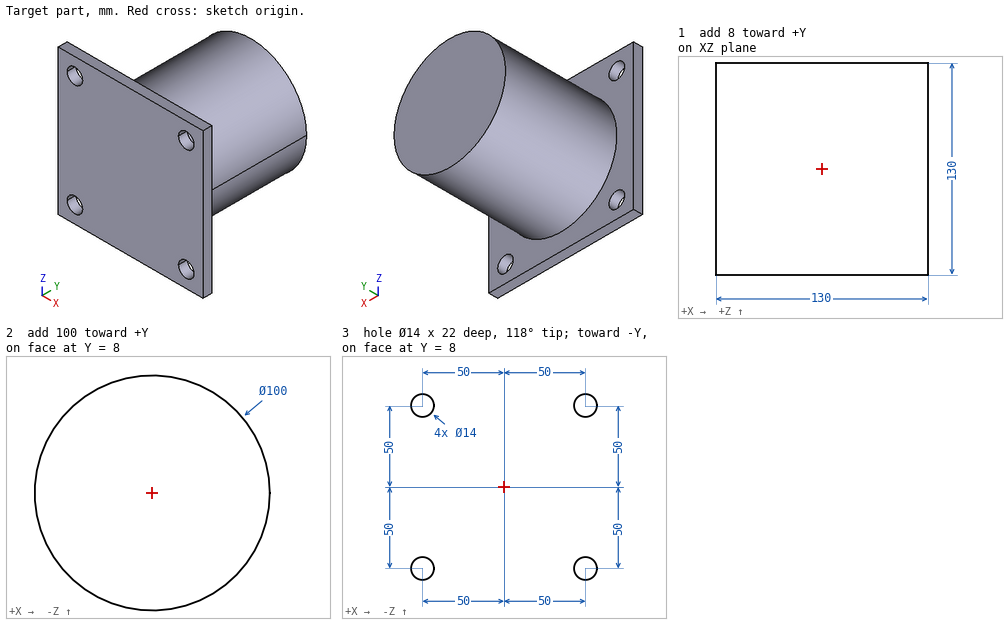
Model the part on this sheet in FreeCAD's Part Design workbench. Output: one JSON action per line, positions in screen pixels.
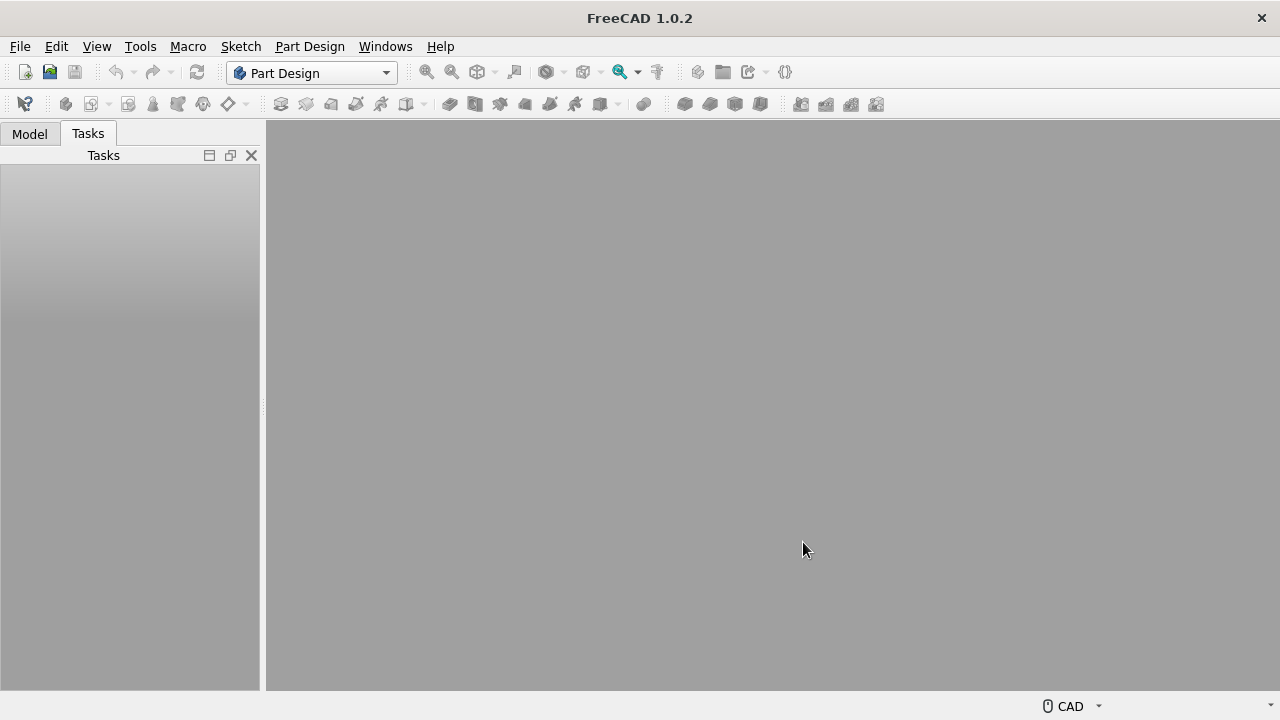
{"action": "left_click", "coordinate": [25, 72]}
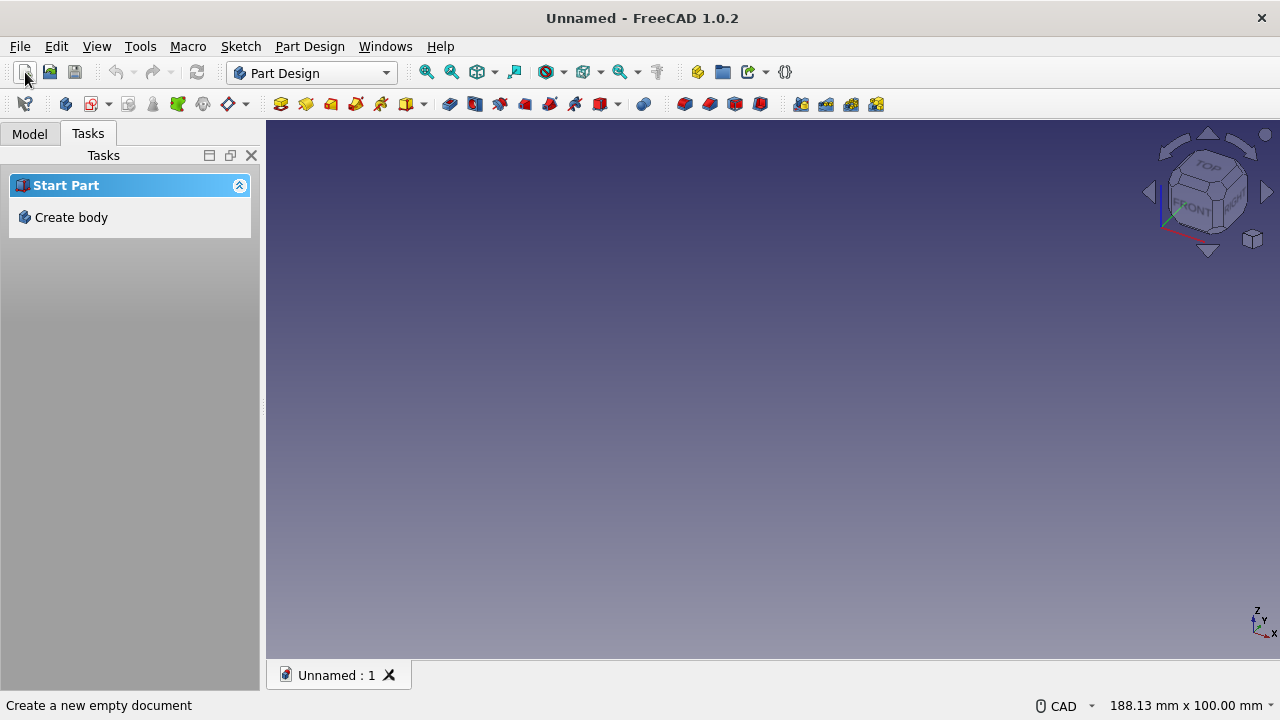
{"action": "left_click", "coordinate": [90, 104]}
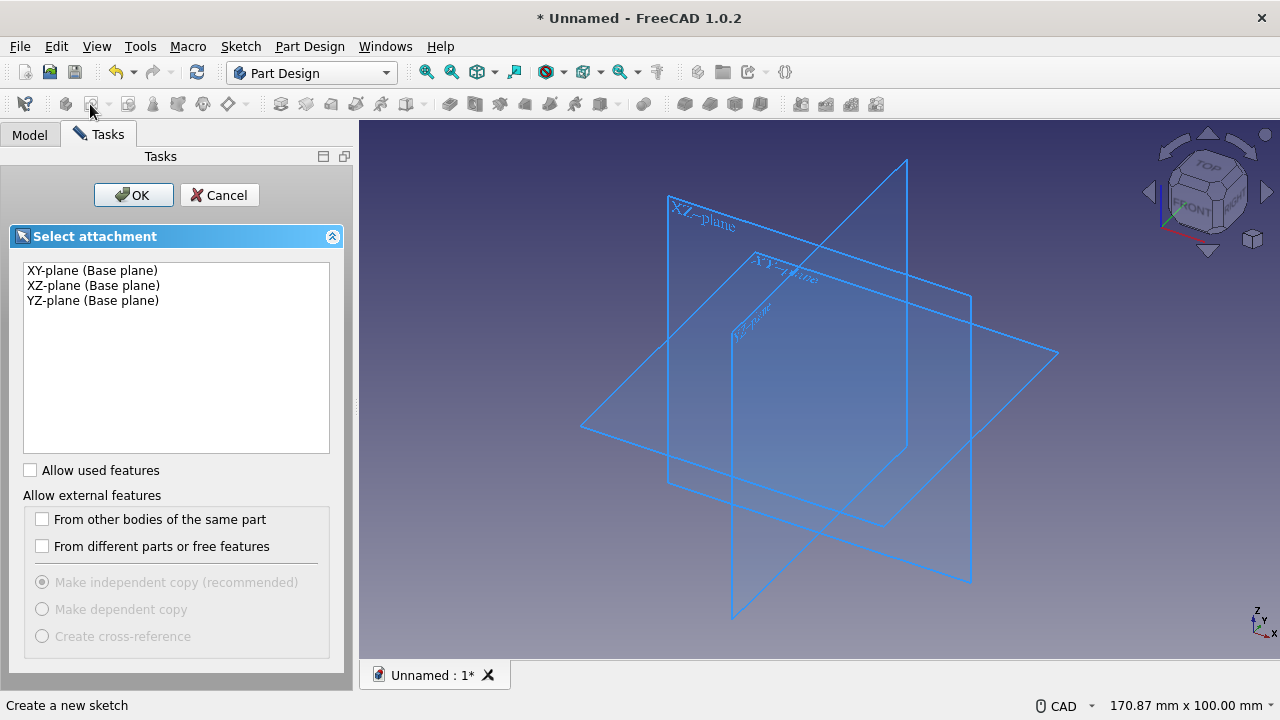
{"action": "left_click", "coordinate": [84, 286]}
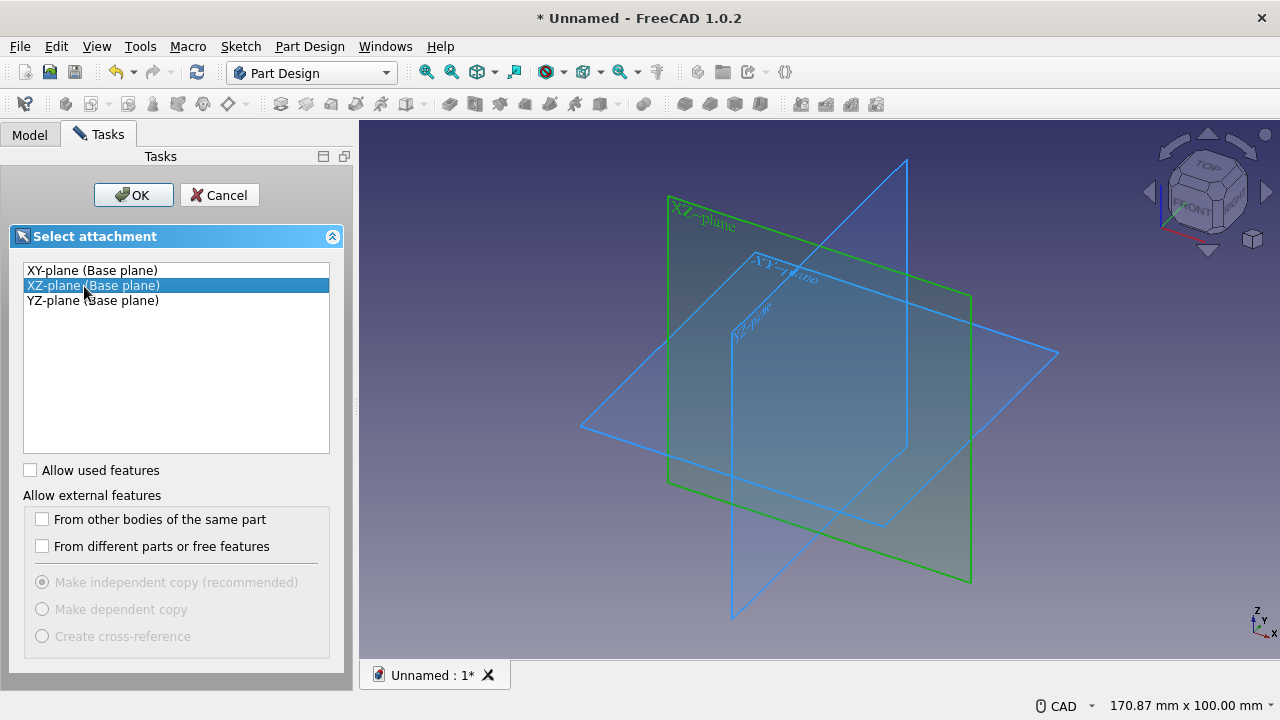
{"action": "left_click", "coordinate": [134, 195]}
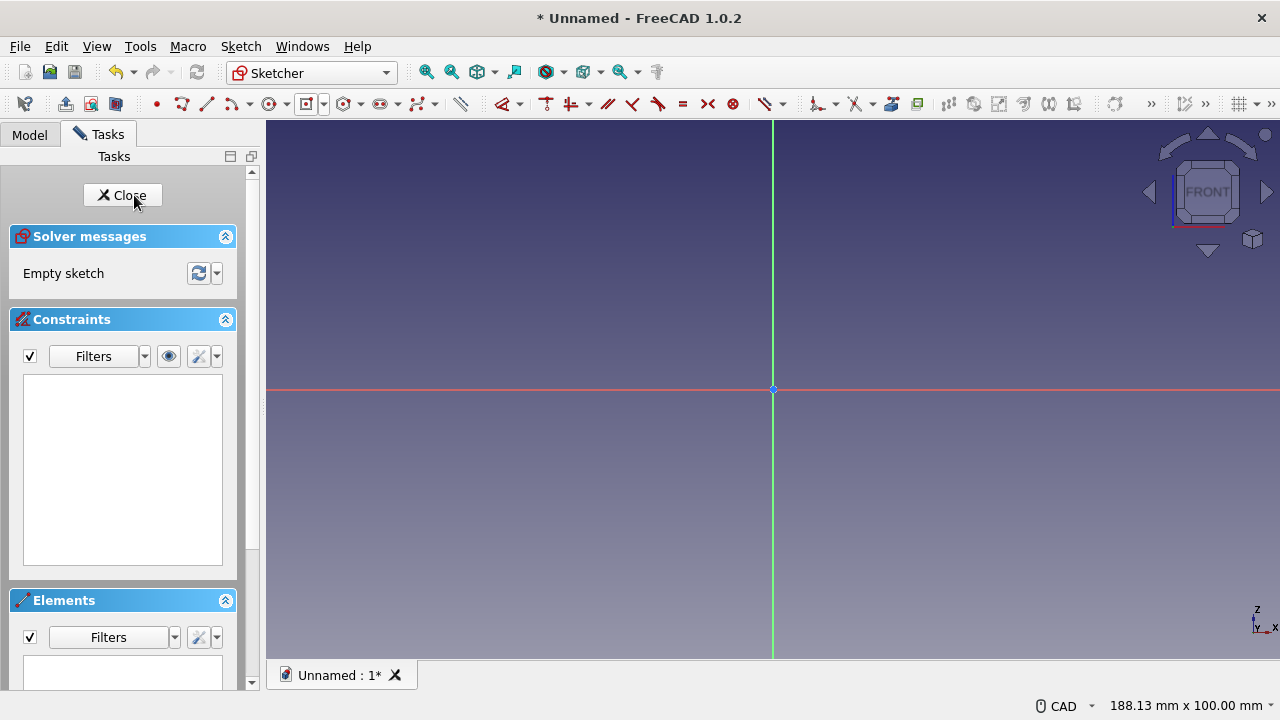
{"action": "scroll", "coordinate": [649, 390], "scroll_direction": "down", "scroll_amount": 4}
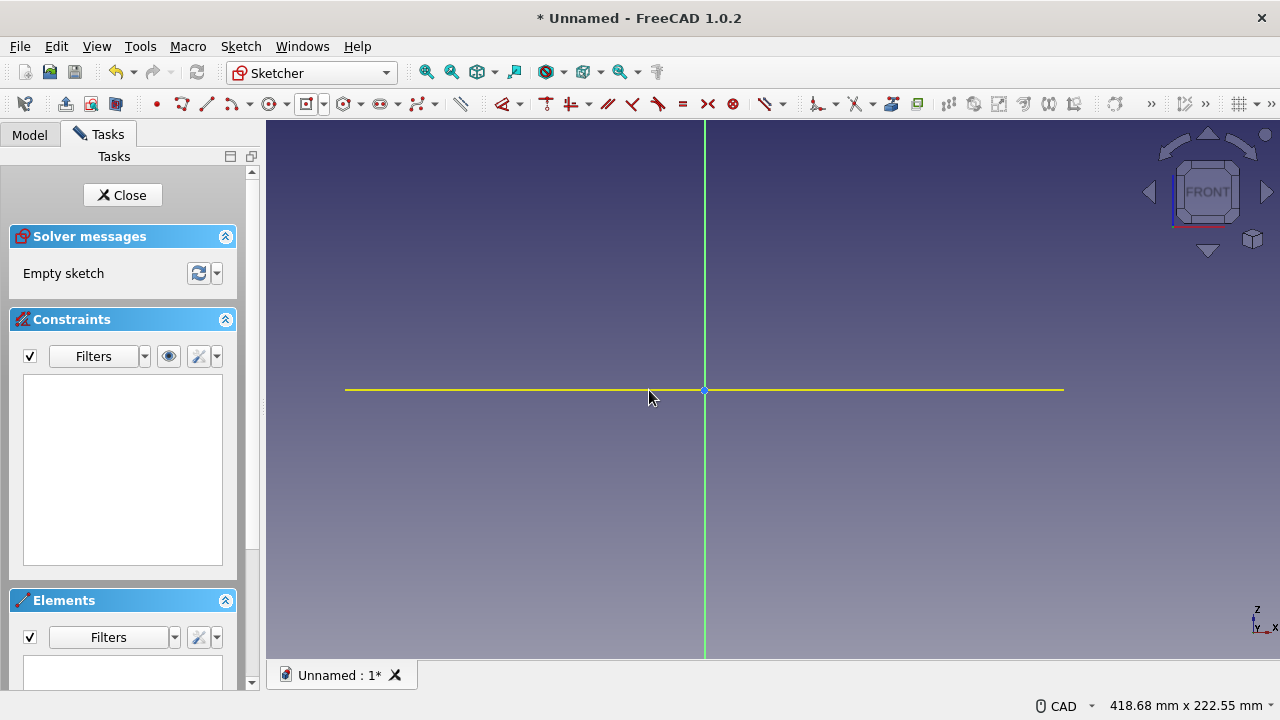
{"action": "left_click", "coordinate": [306, 104]}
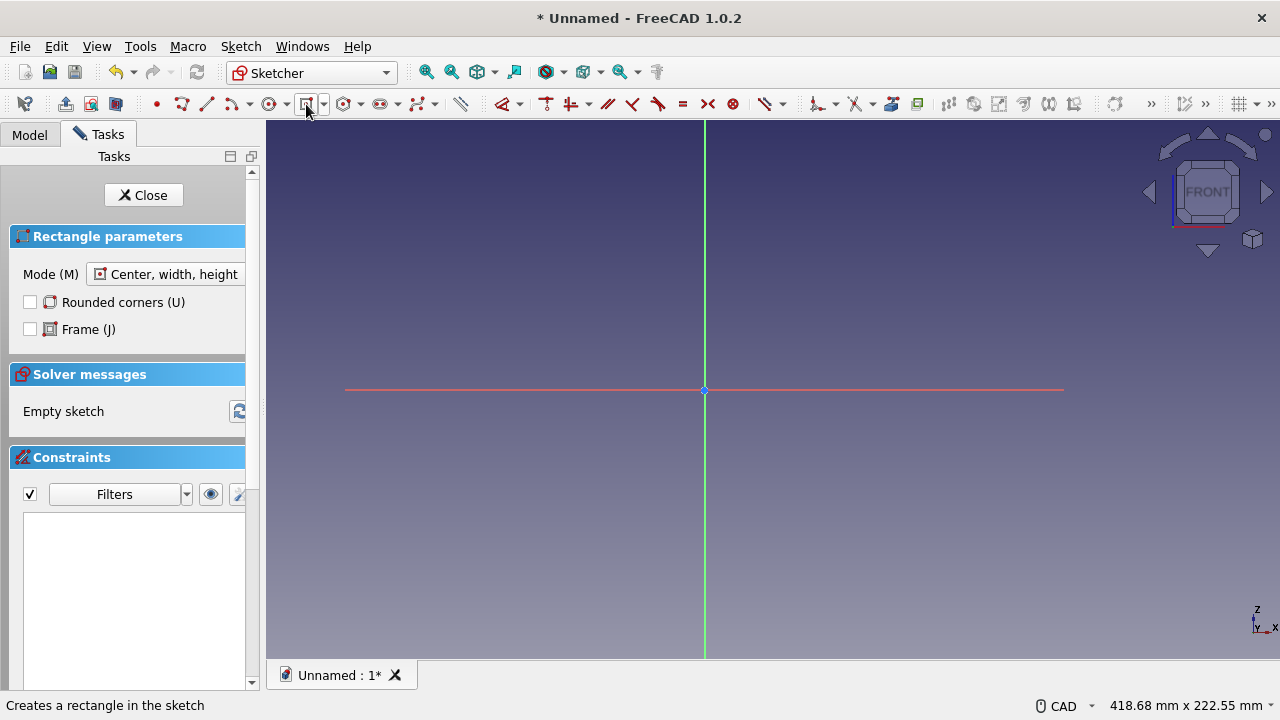
{"action": "left_click", "coordinate": [705, 390]}
{"action": "left_click", "coordinate": [862, 233]}
{"action": "key", "text": "Escape"}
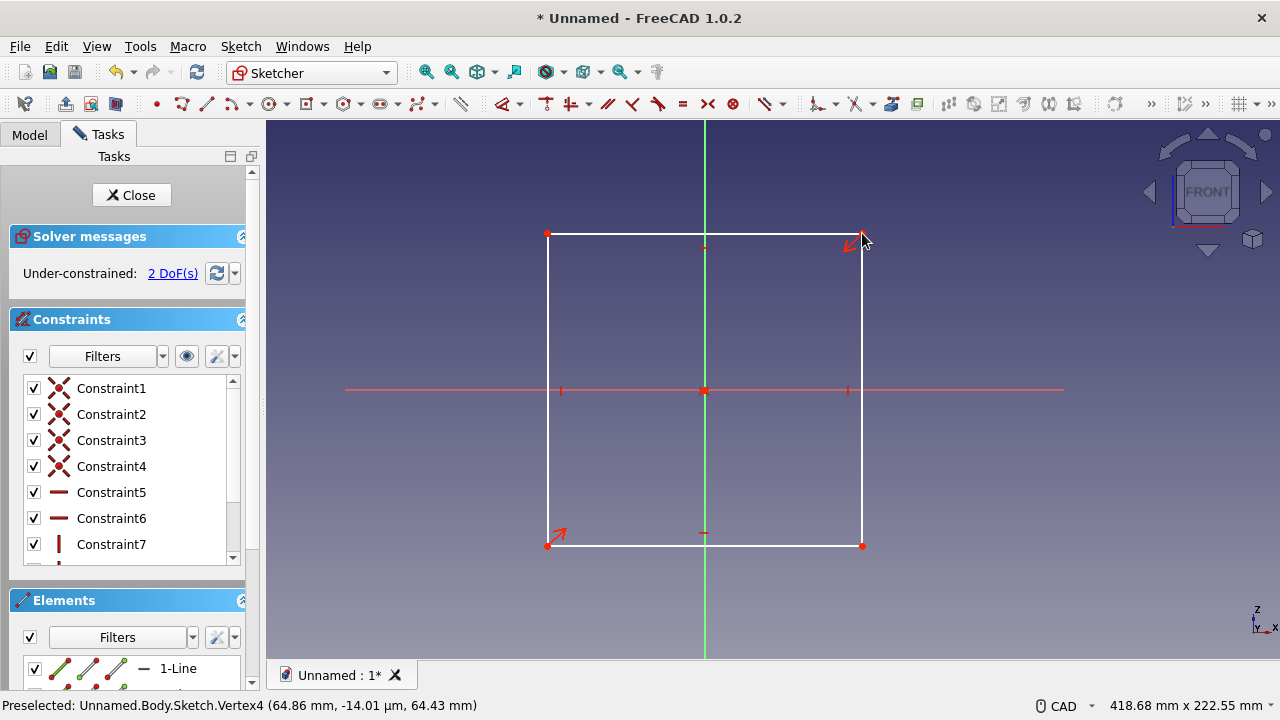
{"action": "left_click", "coordinate": [502, 104]}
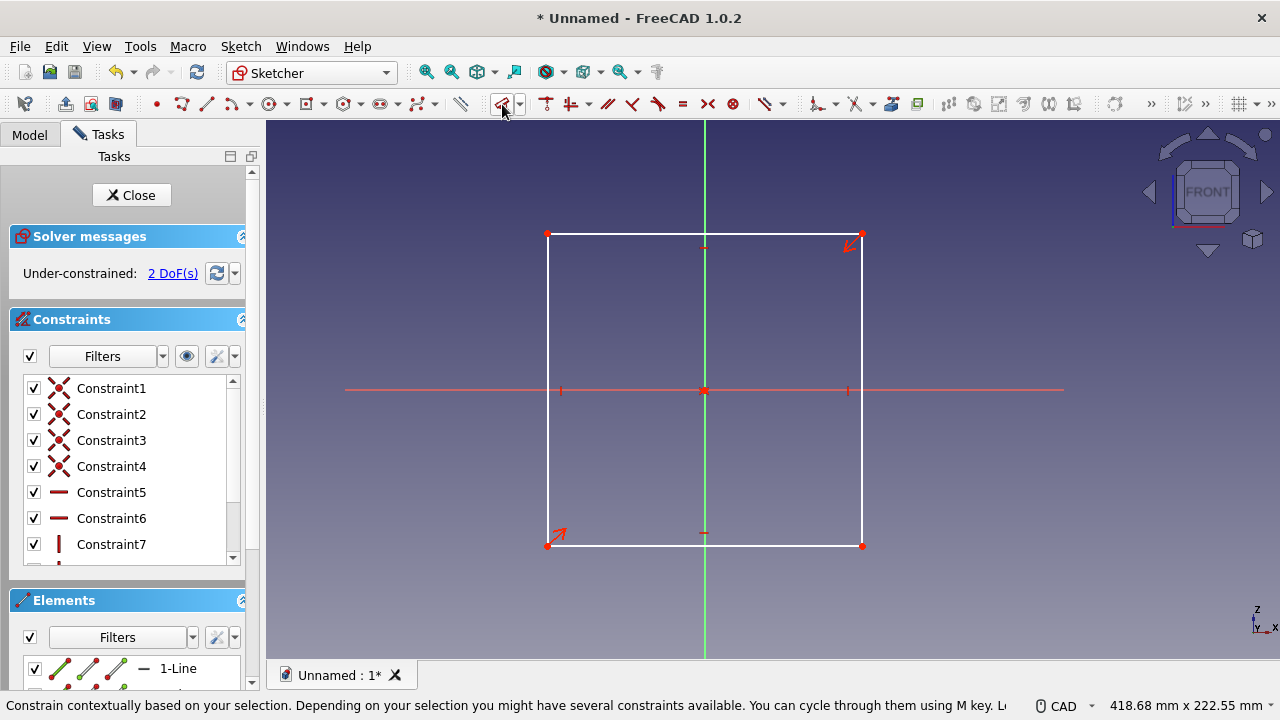
{"action": "left_click", "coordinate": [642, 546]}
{"action": "left_click", "coordinate": [633, 580]}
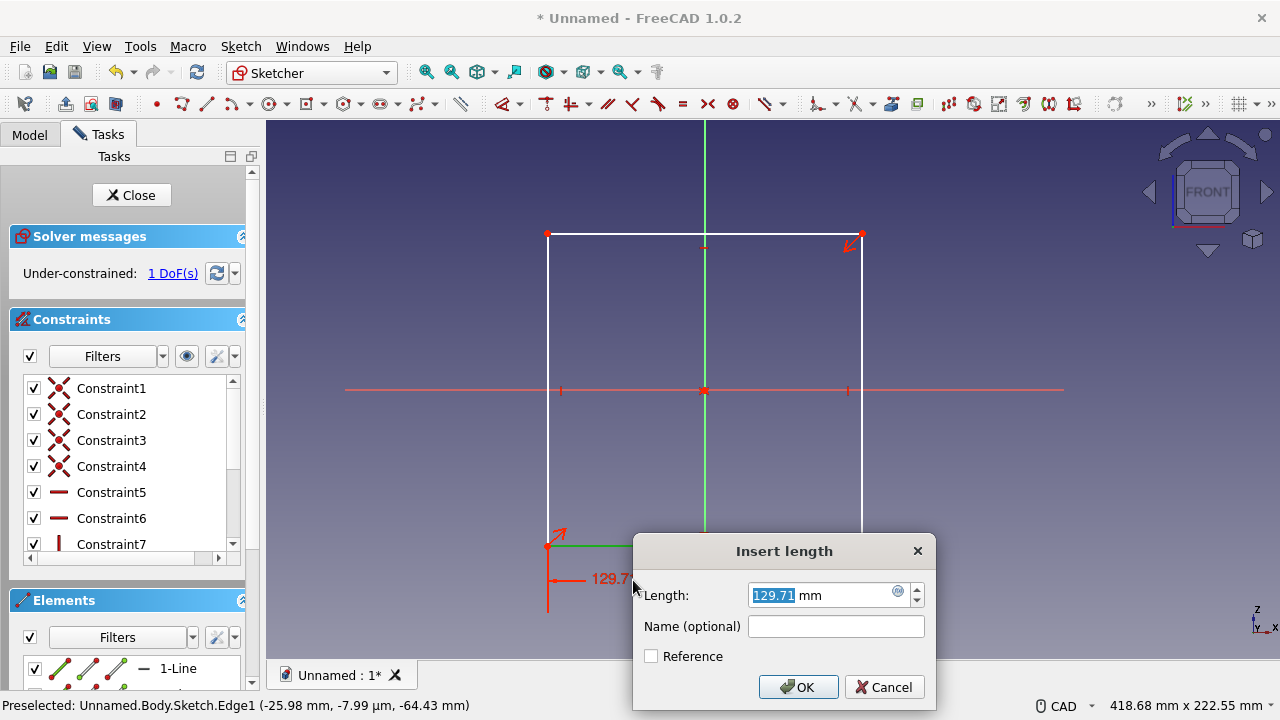
{"action": "type", "text": "130"}
{"action": "key", "text": "Return"}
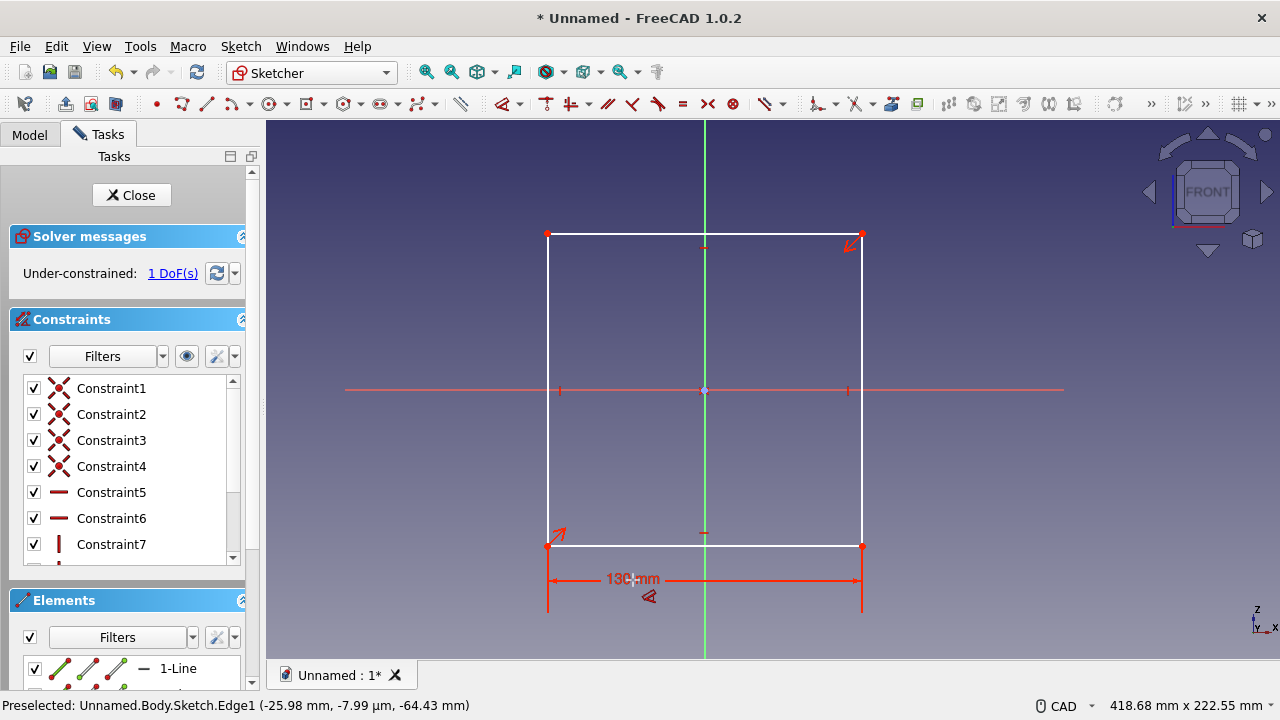
{"action": "left_click", "coordinate": [862, 452]}
{"action": "left_click", "coordinate": [896, 318]}